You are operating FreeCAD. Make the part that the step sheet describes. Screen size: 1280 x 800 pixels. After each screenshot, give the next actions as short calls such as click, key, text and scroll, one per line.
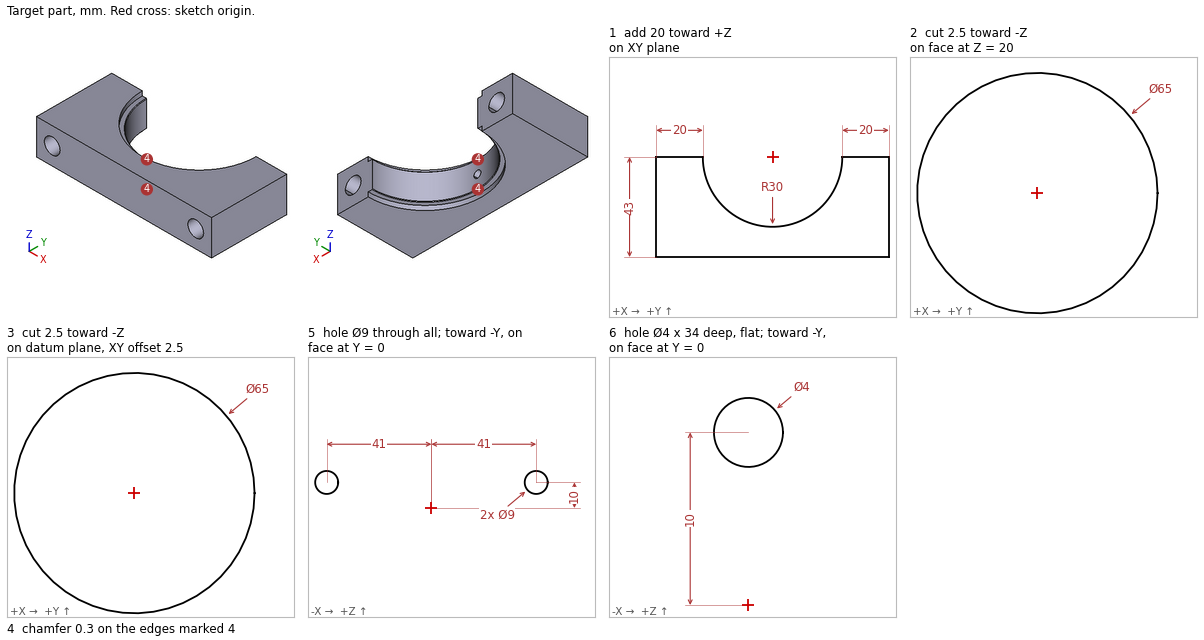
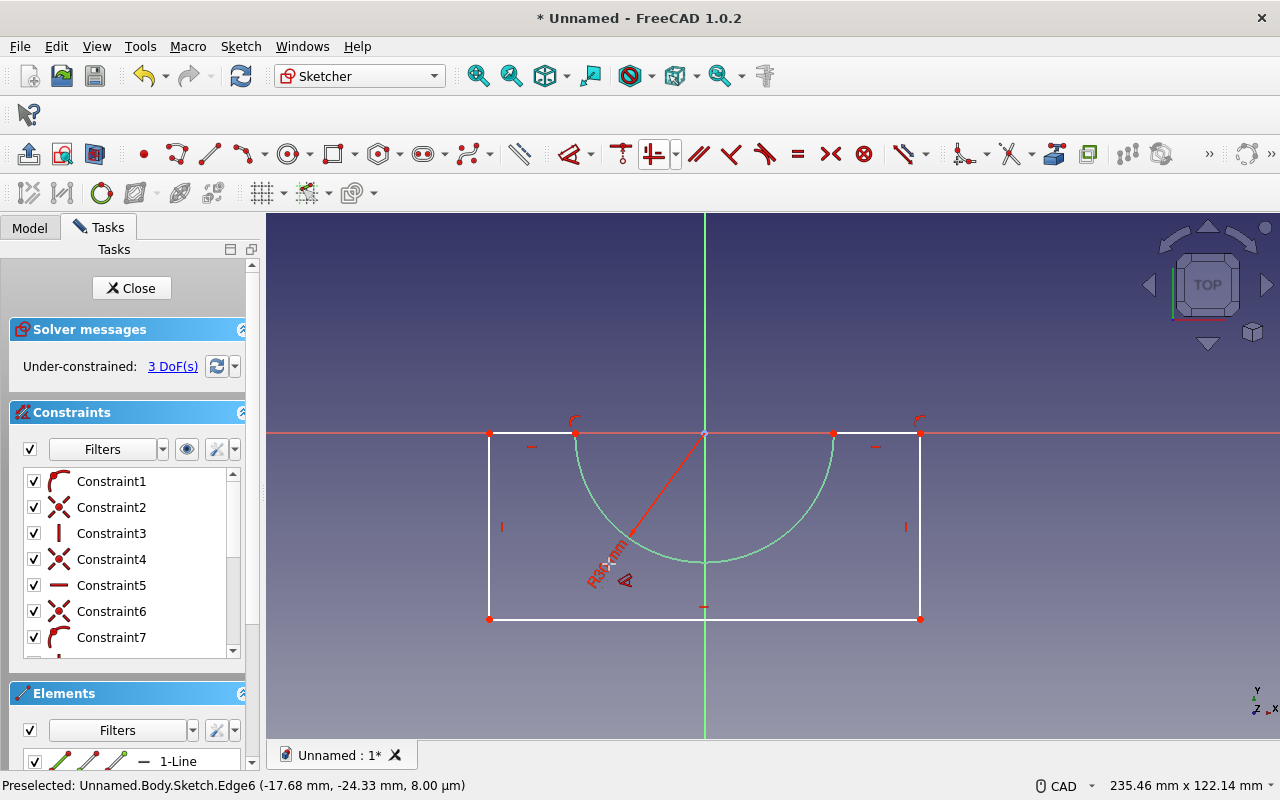
click(549, 433)
click(532, 399)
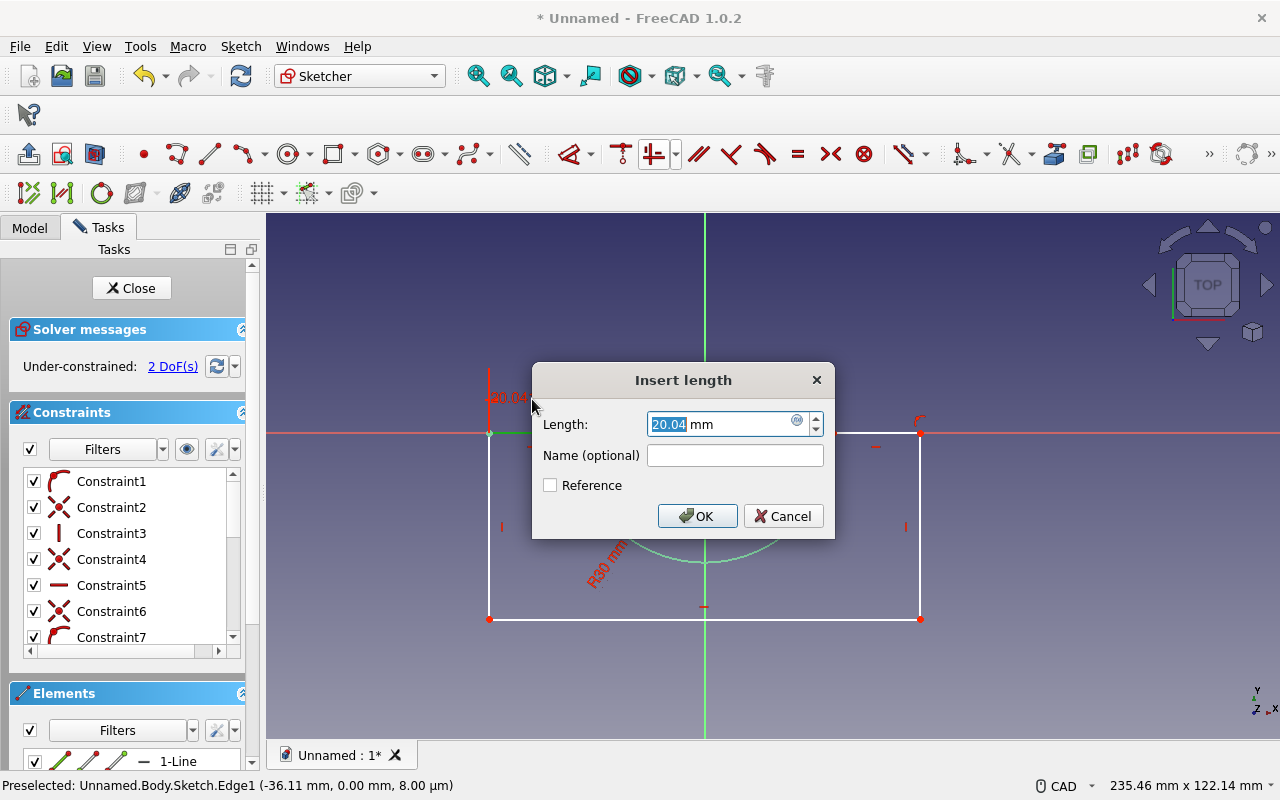
text(20)
key(Return)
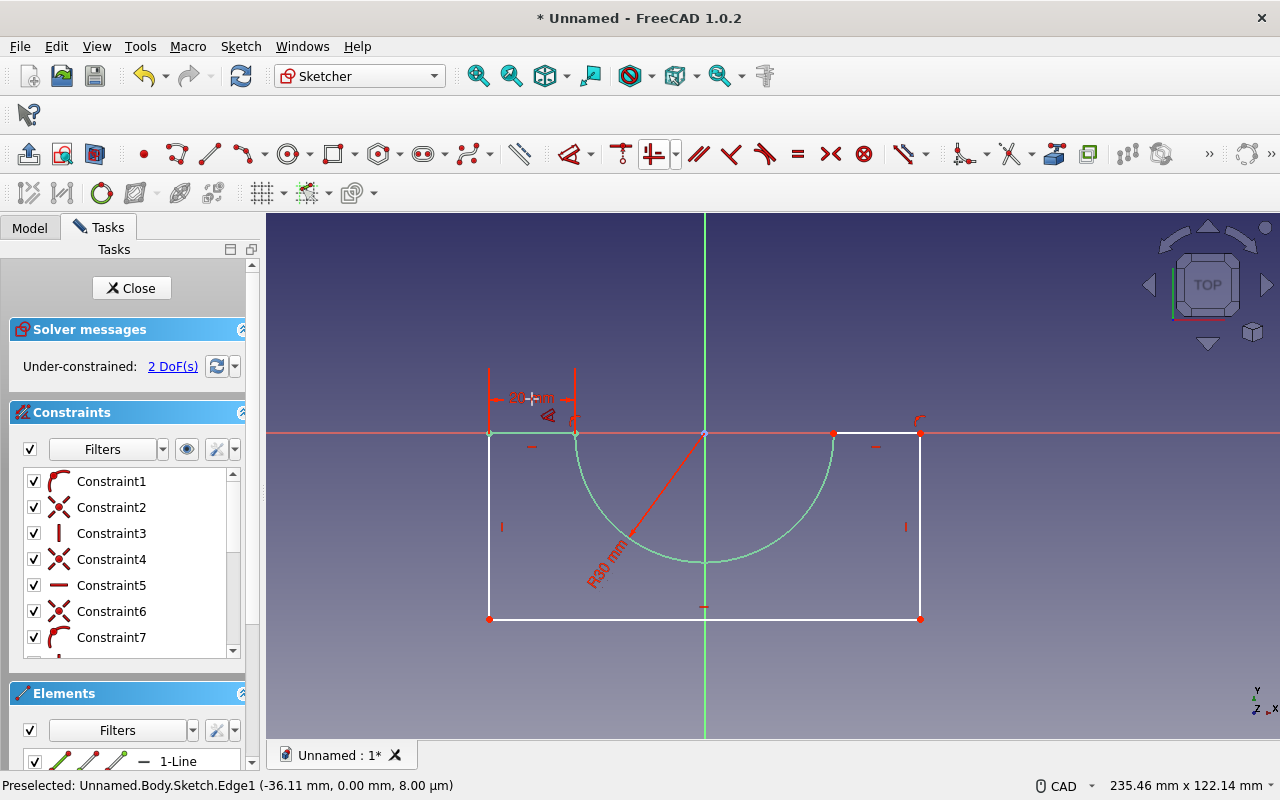
click(489, 489)
click(455, 527)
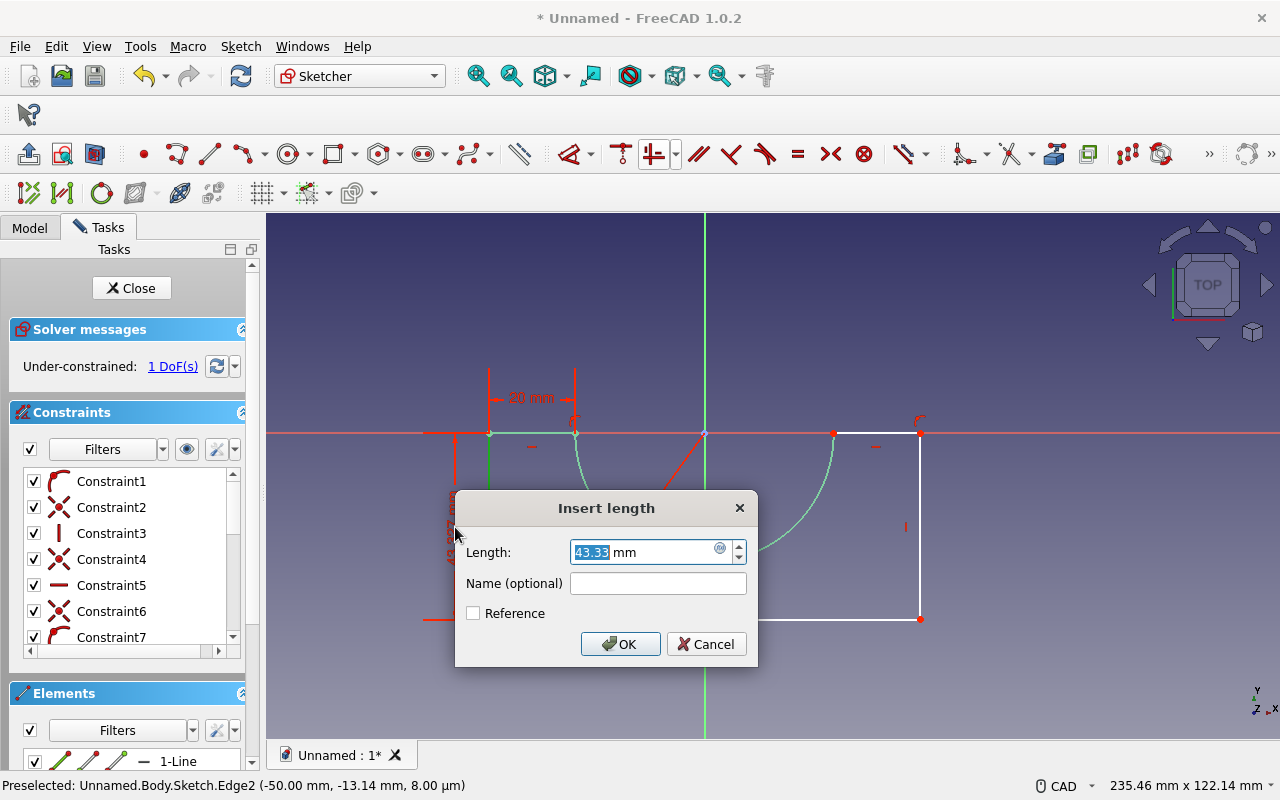
text(43)
key(Return)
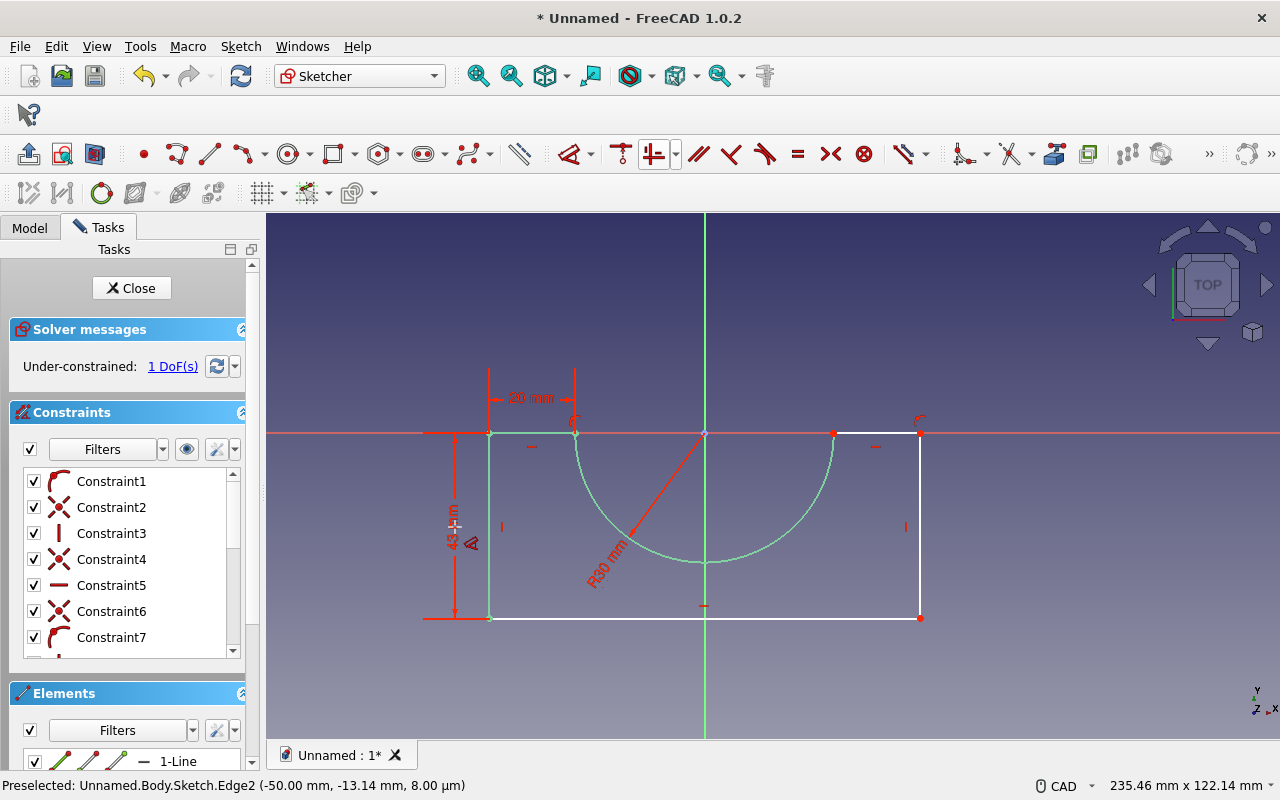
click(894, 433)
click(877, 399)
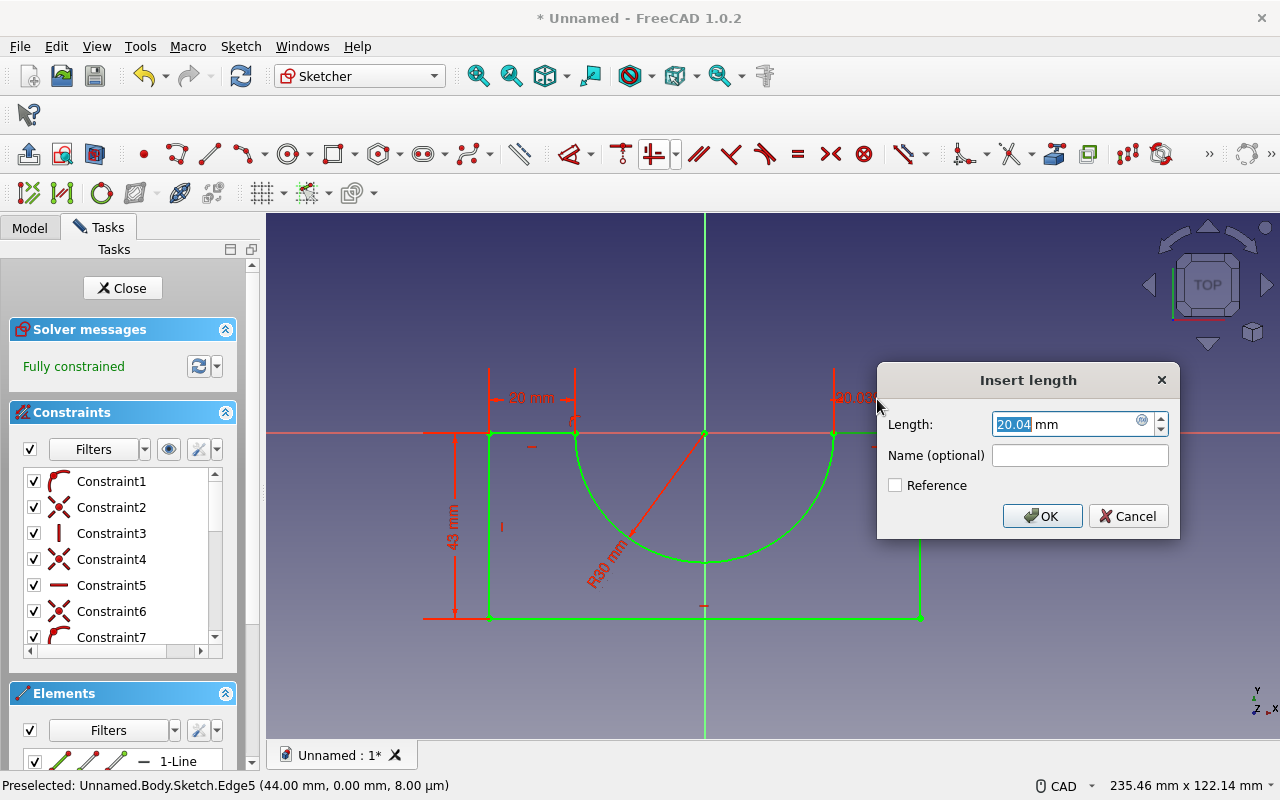
text(20)
key(Return)
key(Escape)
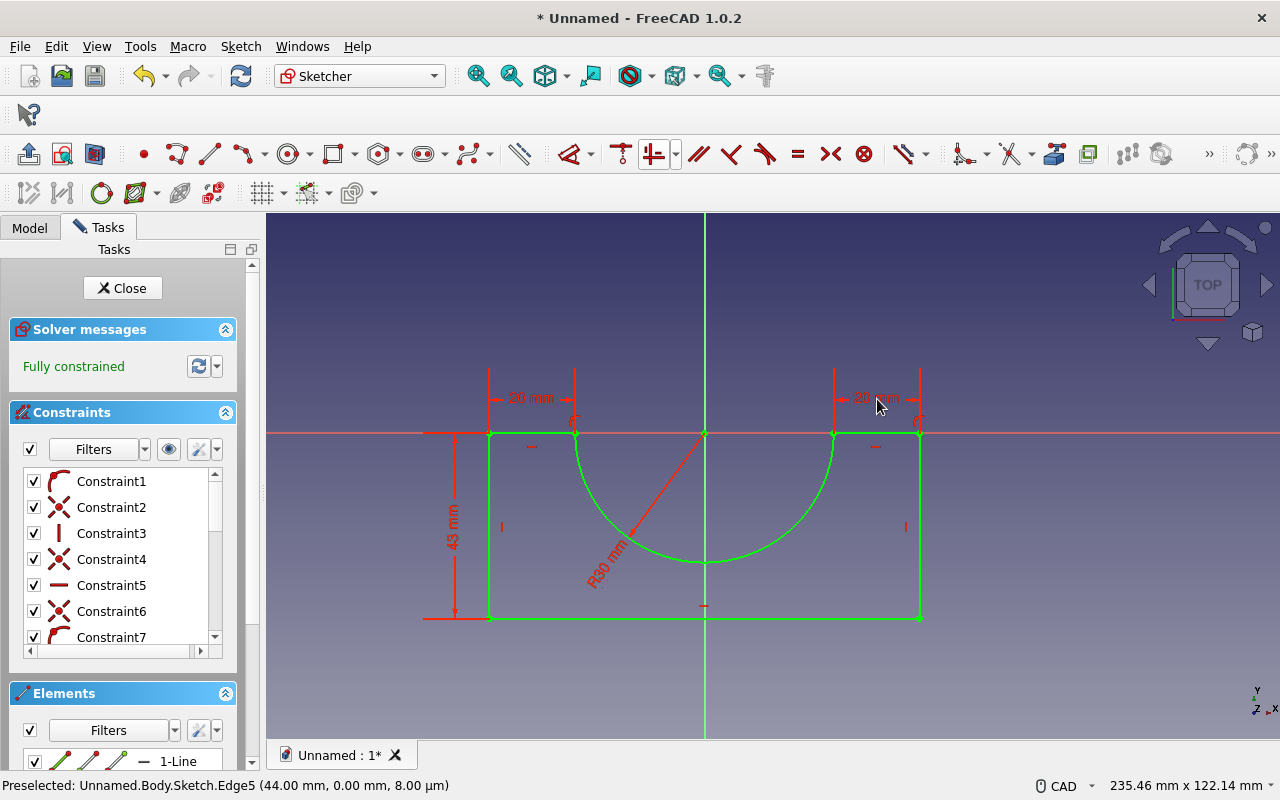
click(123, 288)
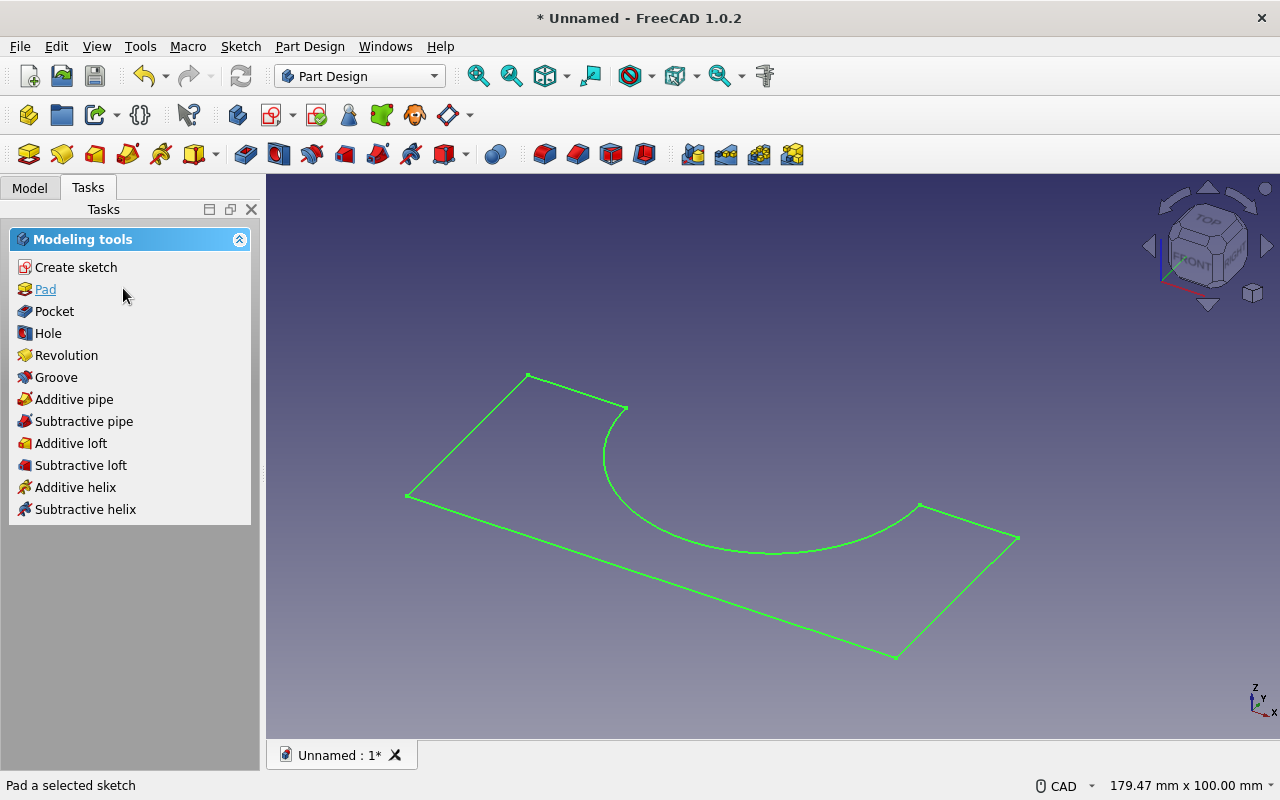
click(29, 154)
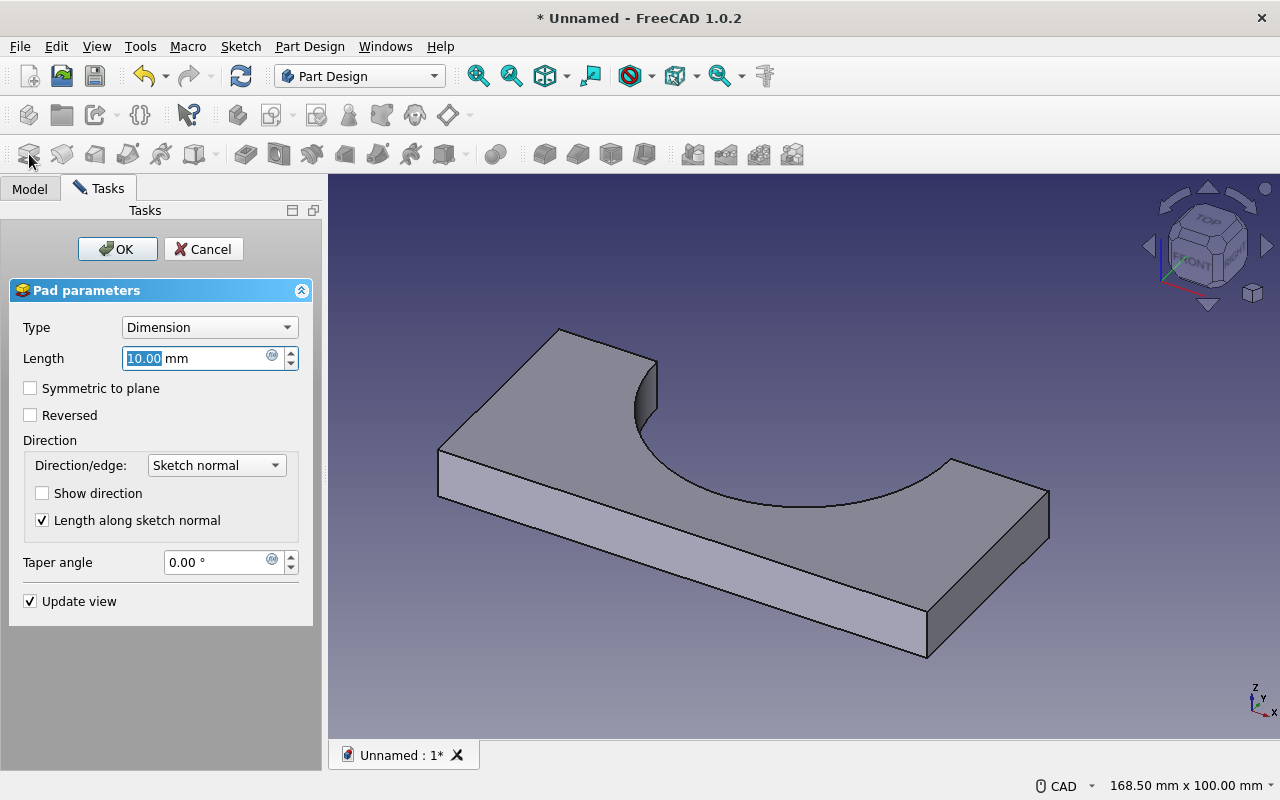
text(20)
key(Tab)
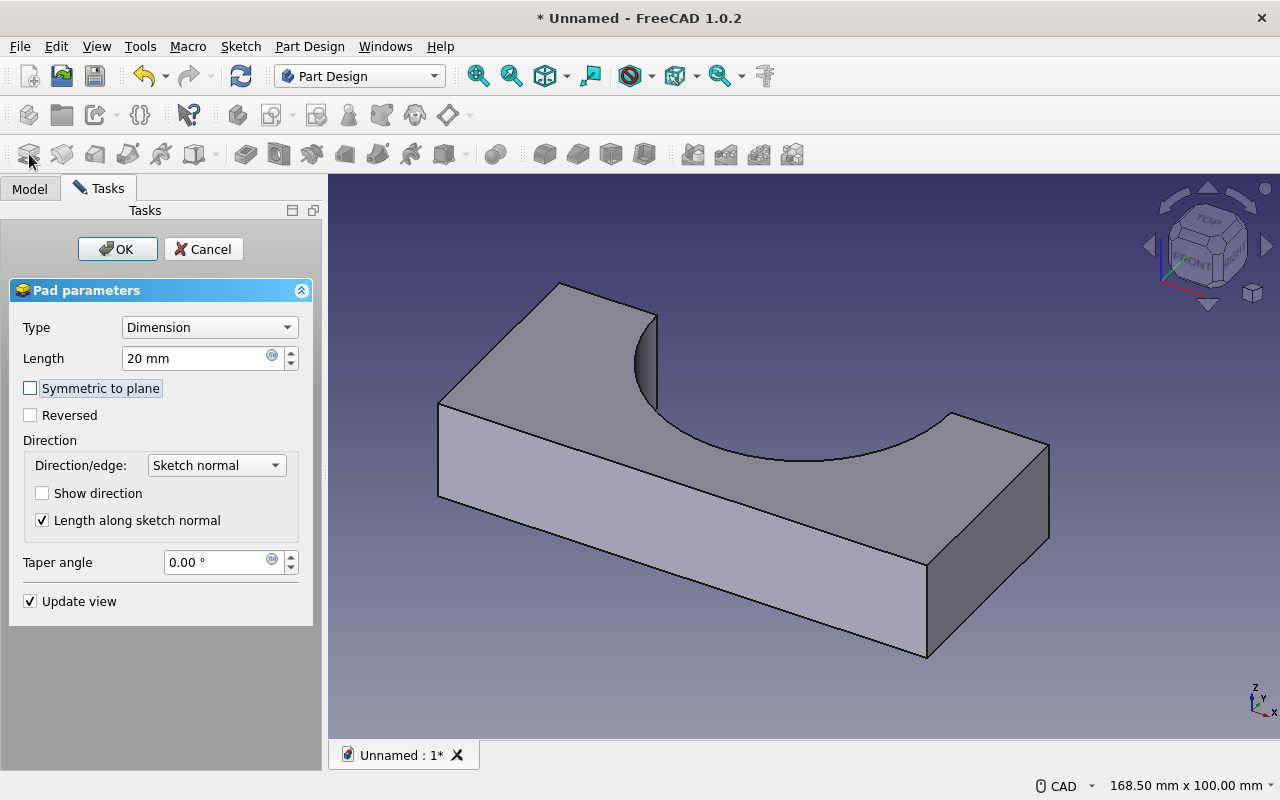
click(118, 249)